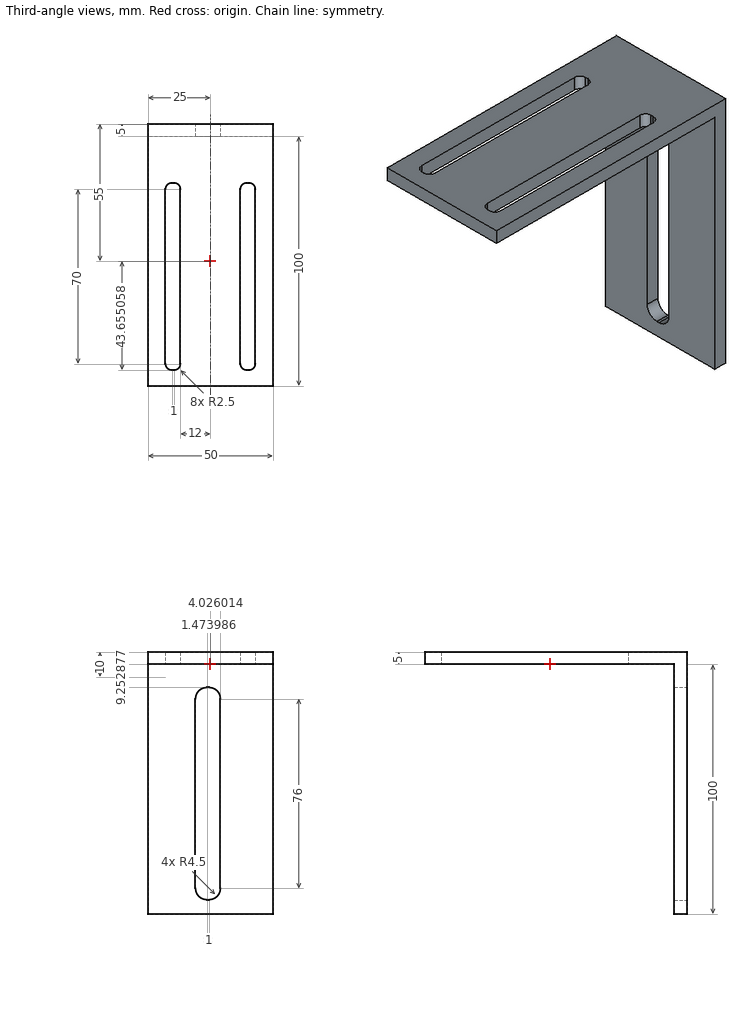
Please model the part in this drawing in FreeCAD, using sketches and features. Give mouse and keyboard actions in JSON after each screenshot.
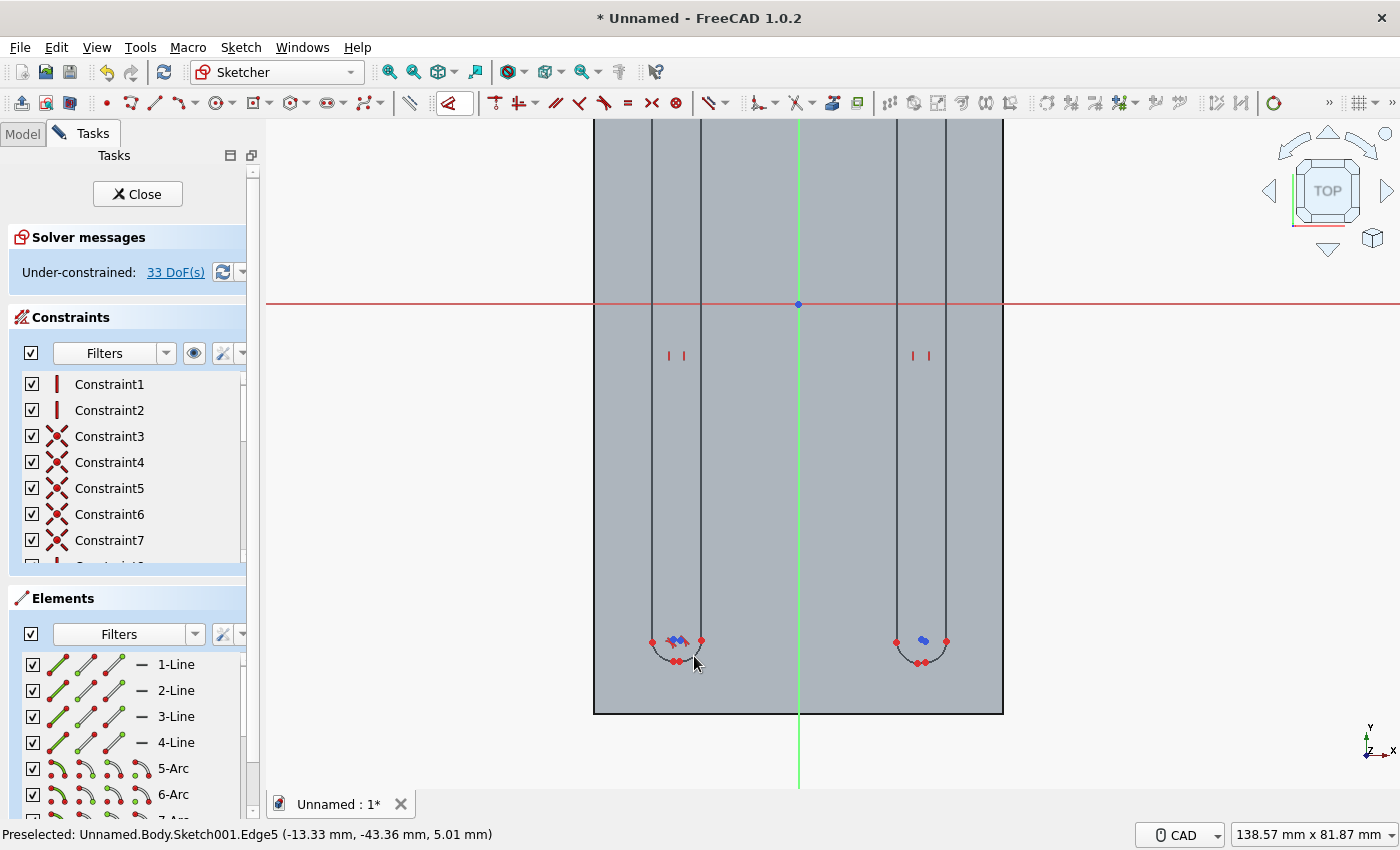
{"action": "left_click", "coordinate": [701, 470]}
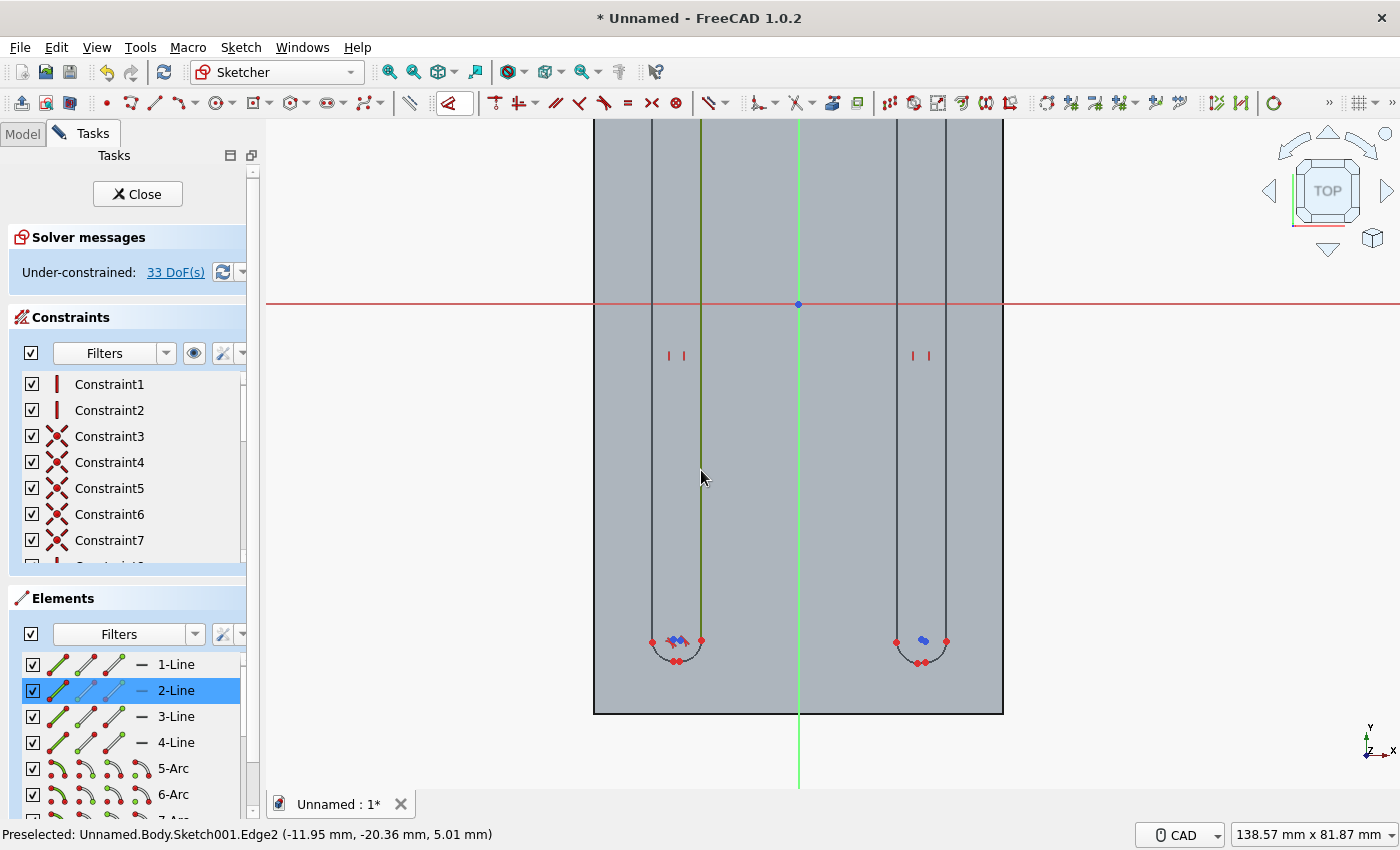
{"action": "scroll", "coordinate": [695, 656], "scroll_direction": "down", "scroll_amount": 2}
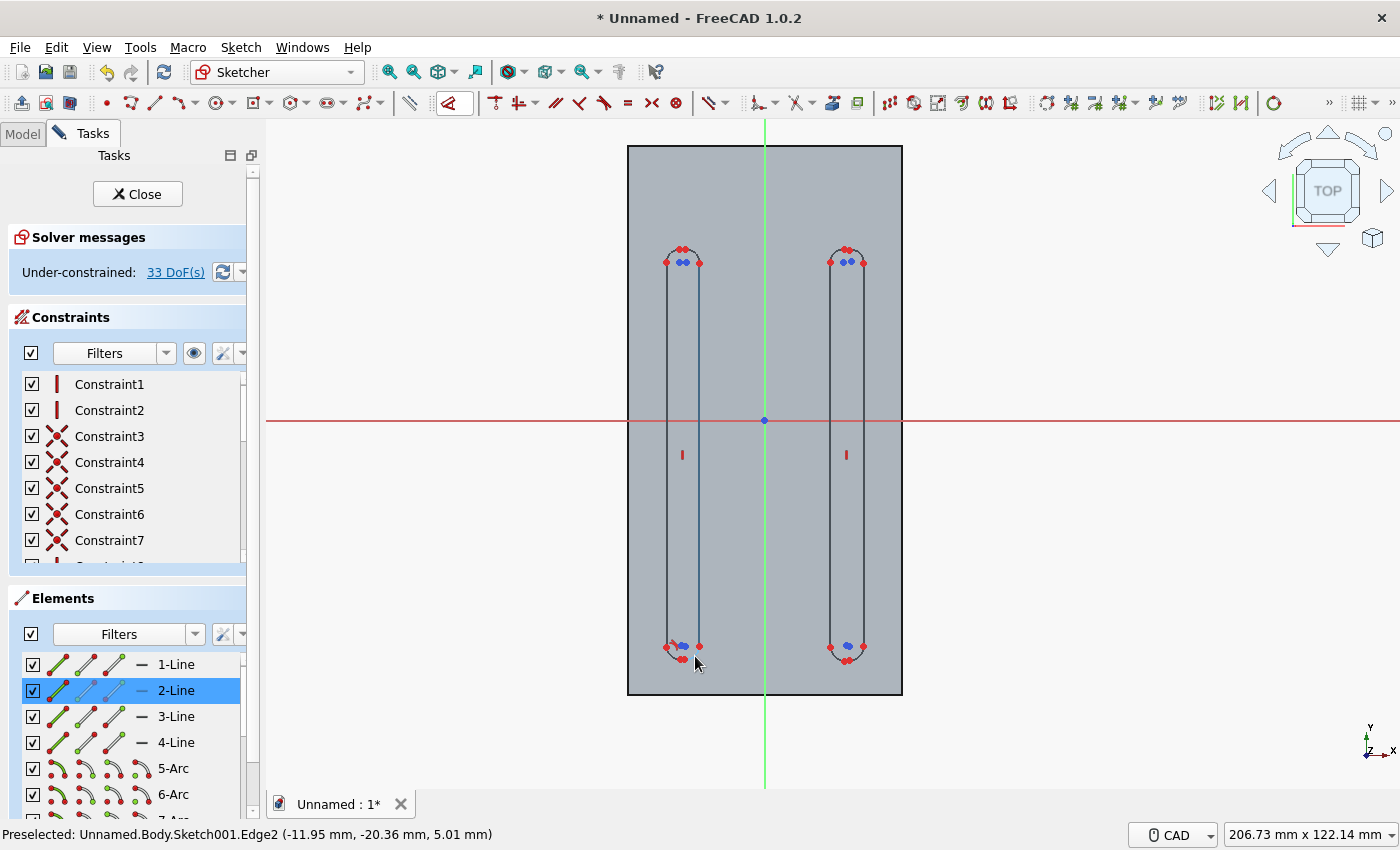
{"action": "scroll", "coordinate": [698, 257], "scroll_direction": "up", "scroll_amount": 4}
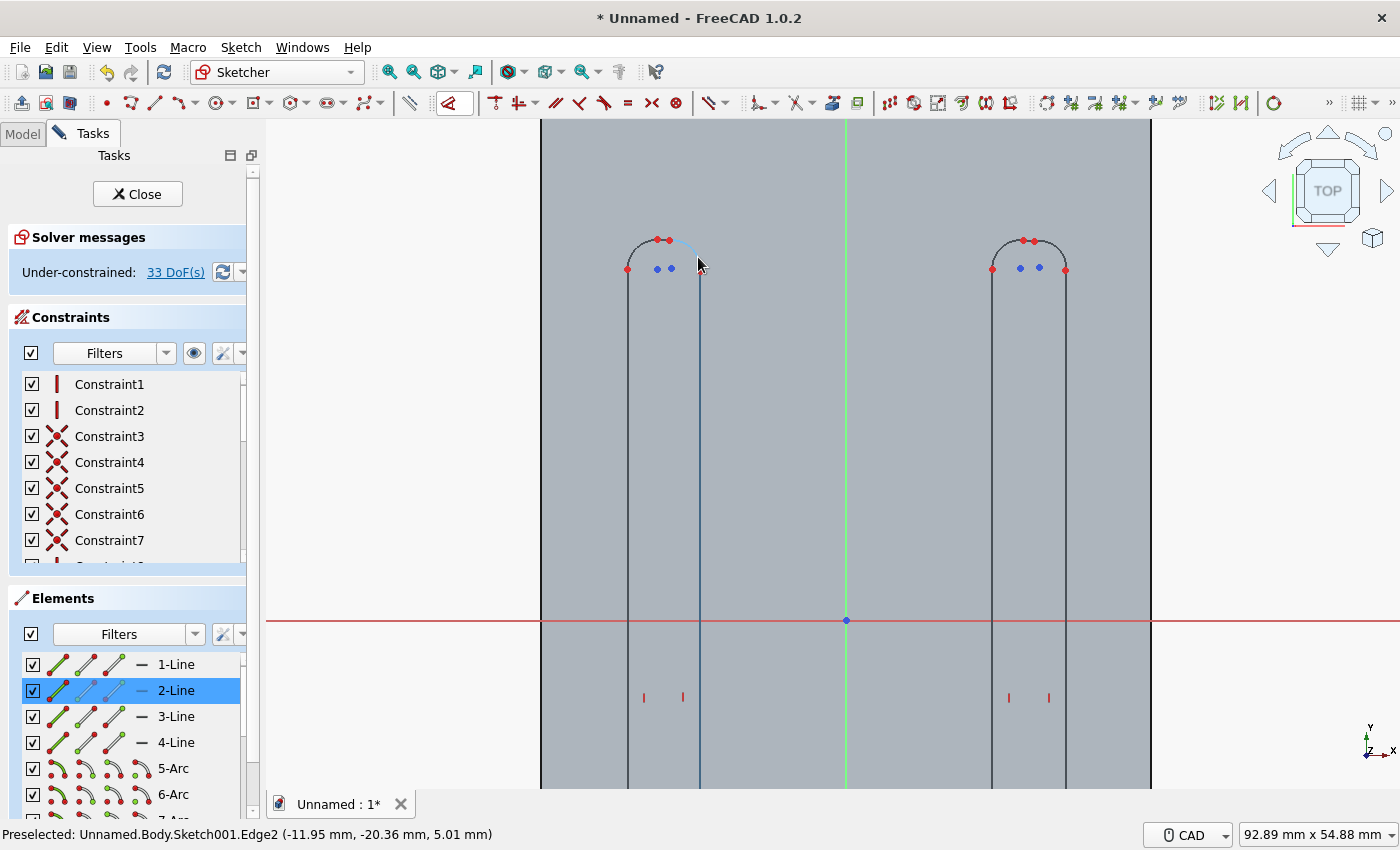
{"action": "left_click", "coordinate": [698, 257]}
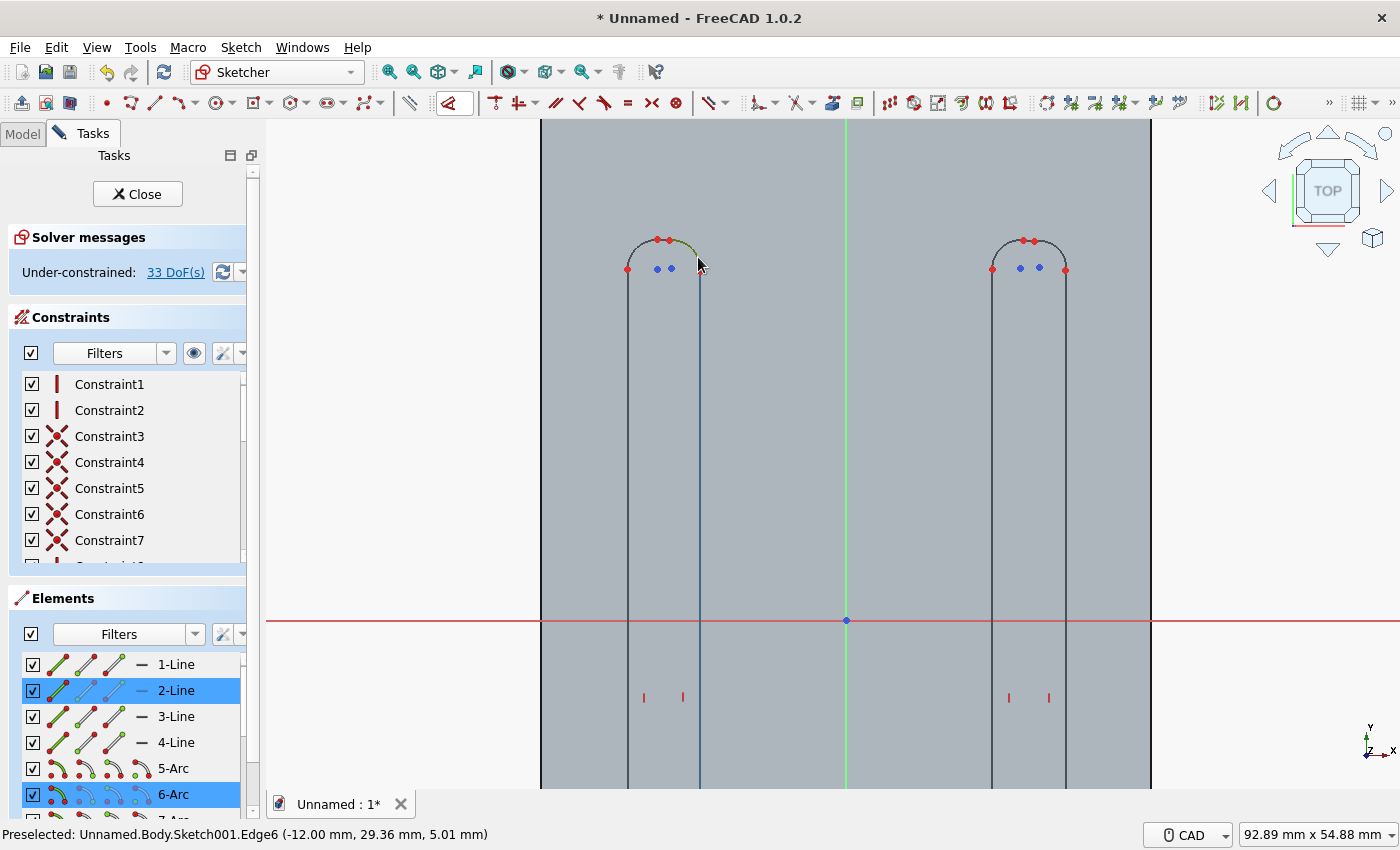
{"action": "left_click", "coordinate": [604, 104]}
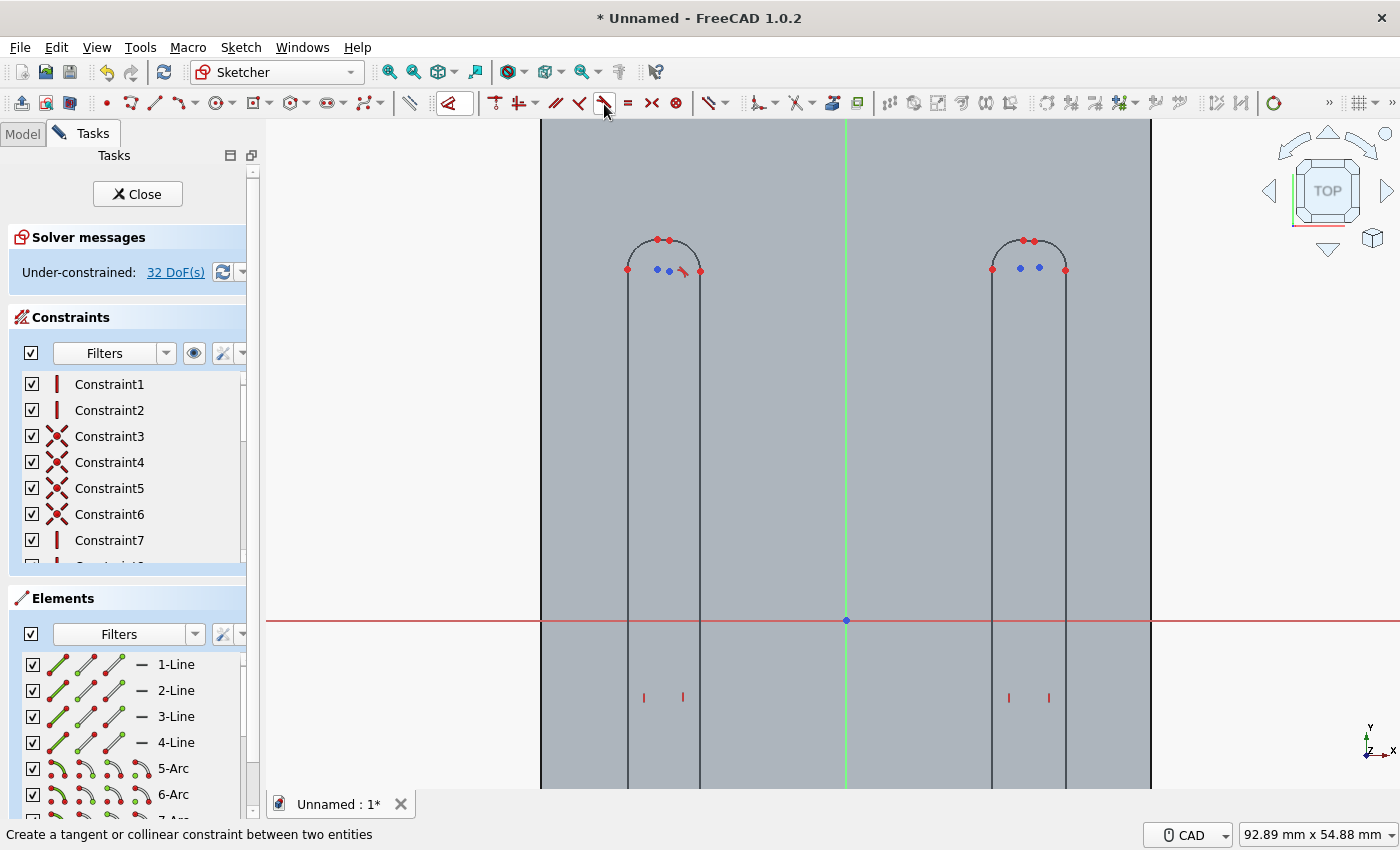
{"action": "scroll", "coordinate": [663, 240], "scroll_direction": "up", "scroll_amount": 5}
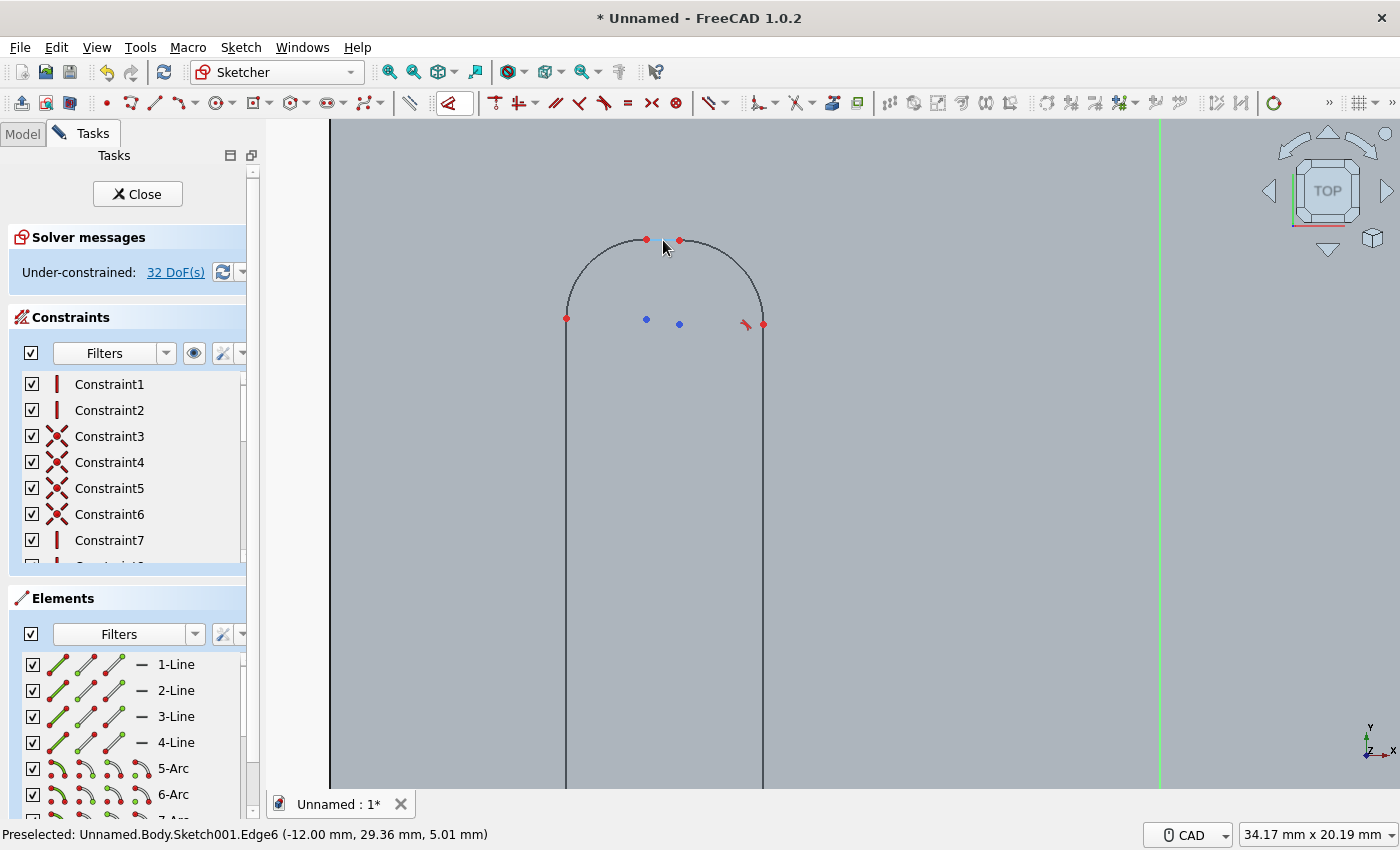
{"action": "left_click", "coordinate": [663, 240]}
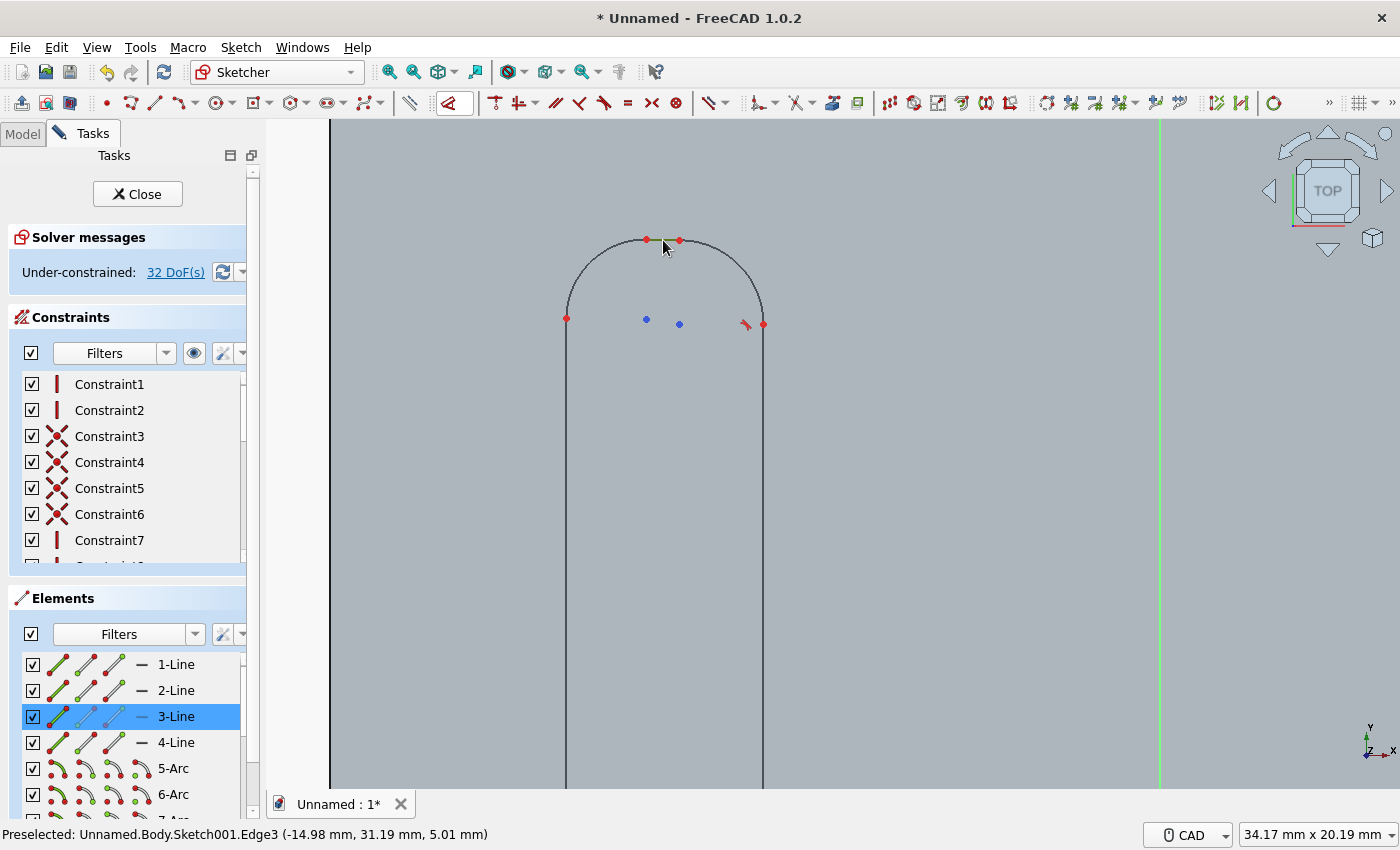
{"action": "left_click", "coordinate": [754, 286]}